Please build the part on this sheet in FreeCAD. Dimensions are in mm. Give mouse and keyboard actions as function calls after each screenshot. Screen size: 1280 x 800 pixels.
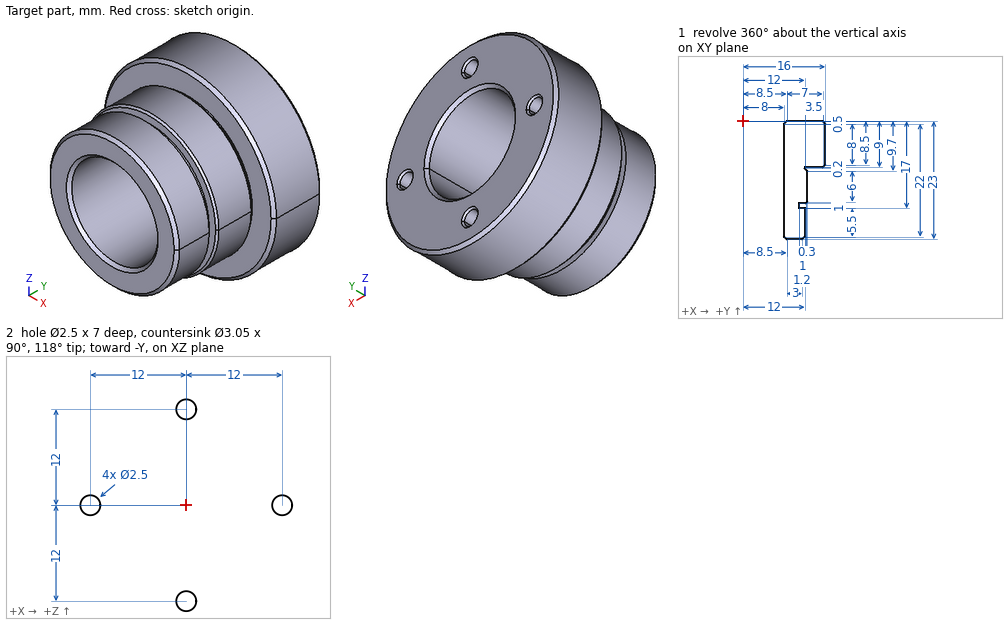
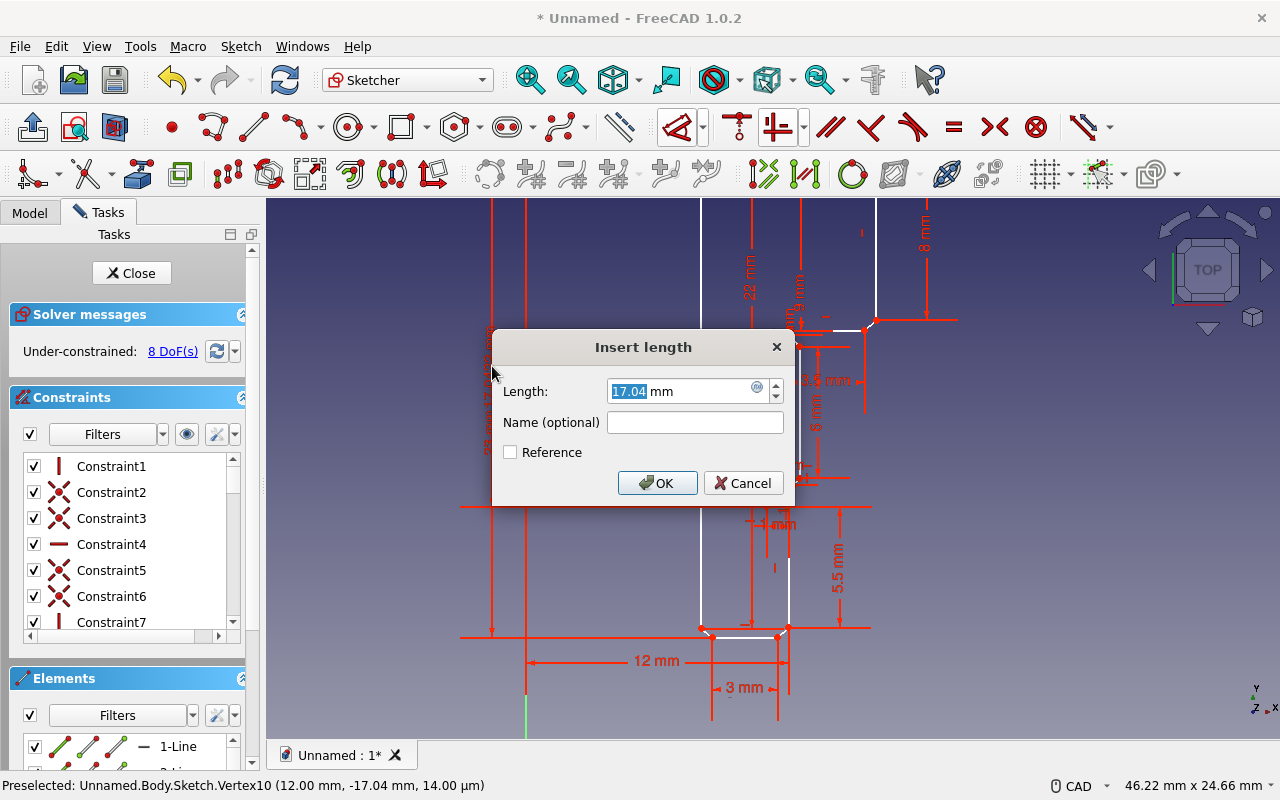
text(17)
key(Return)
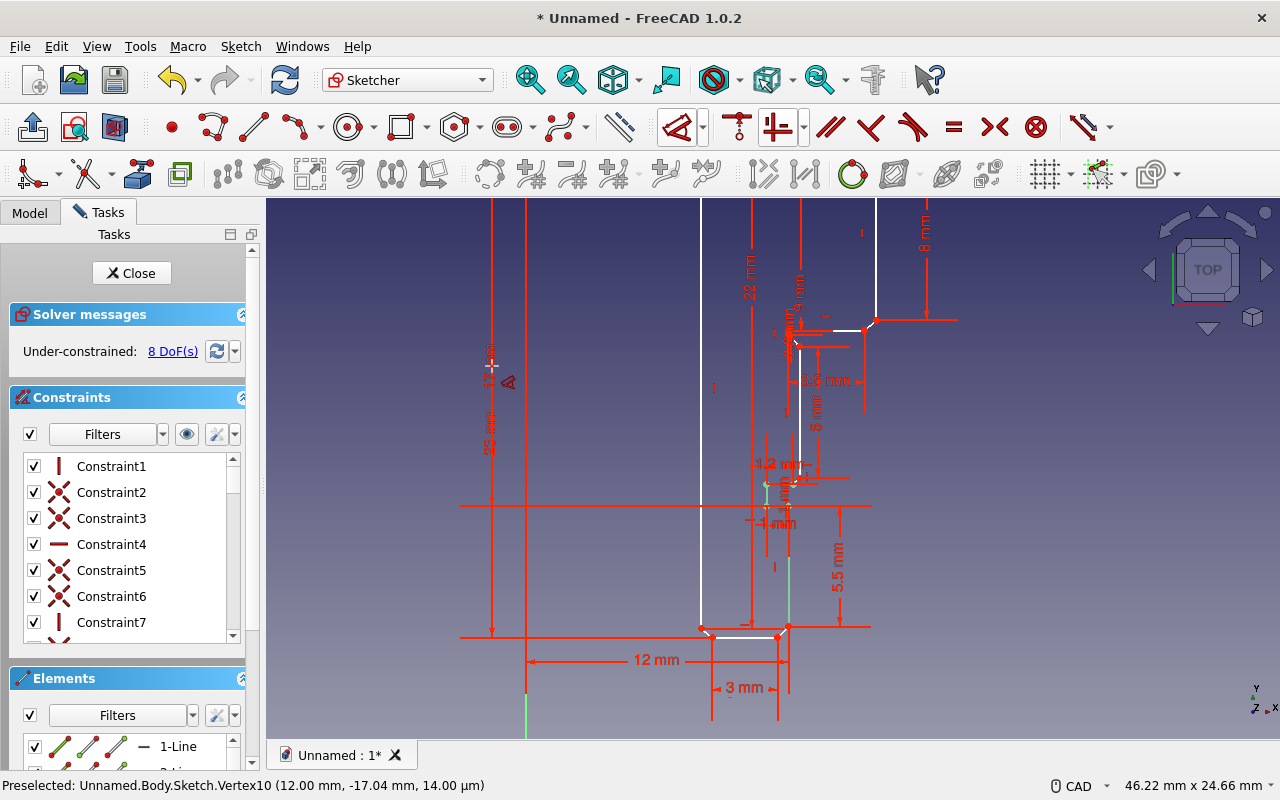
scroll(788, 335, up, 6)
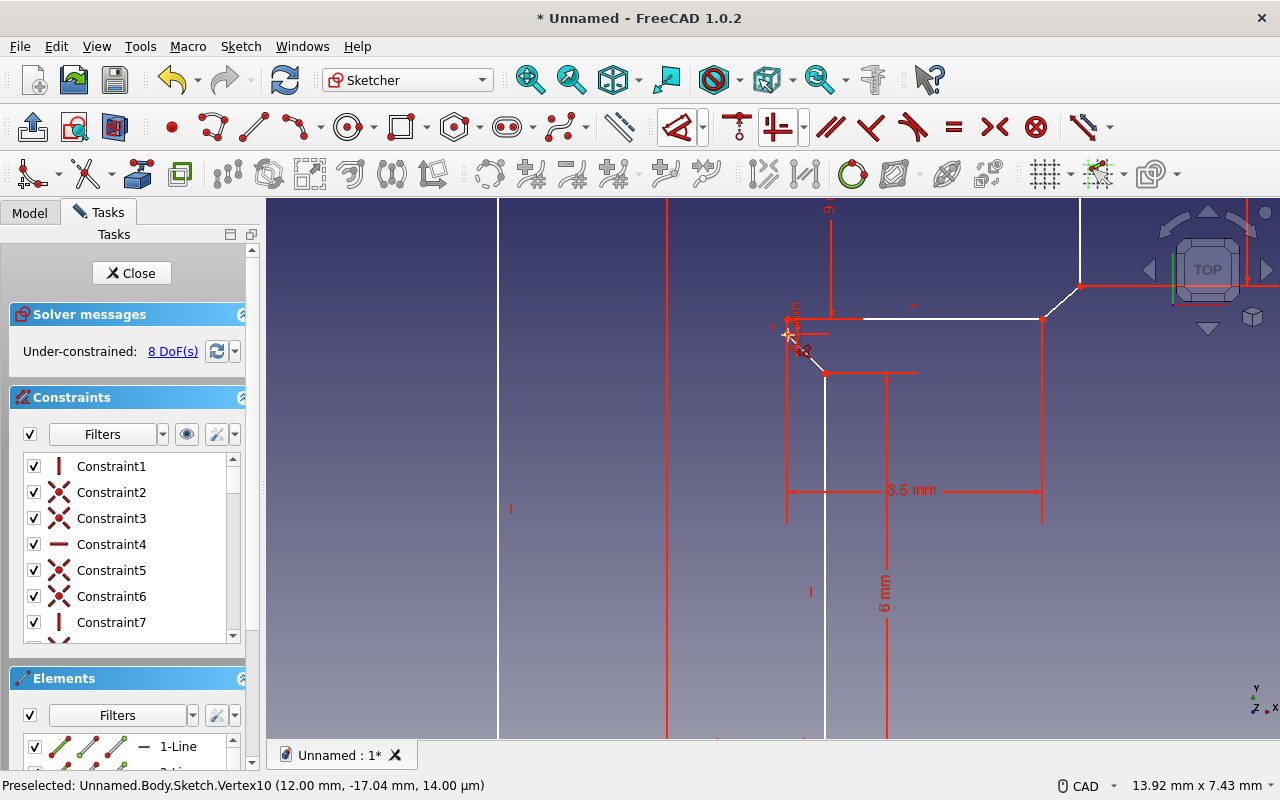
click(787, 334)
click(541, 368)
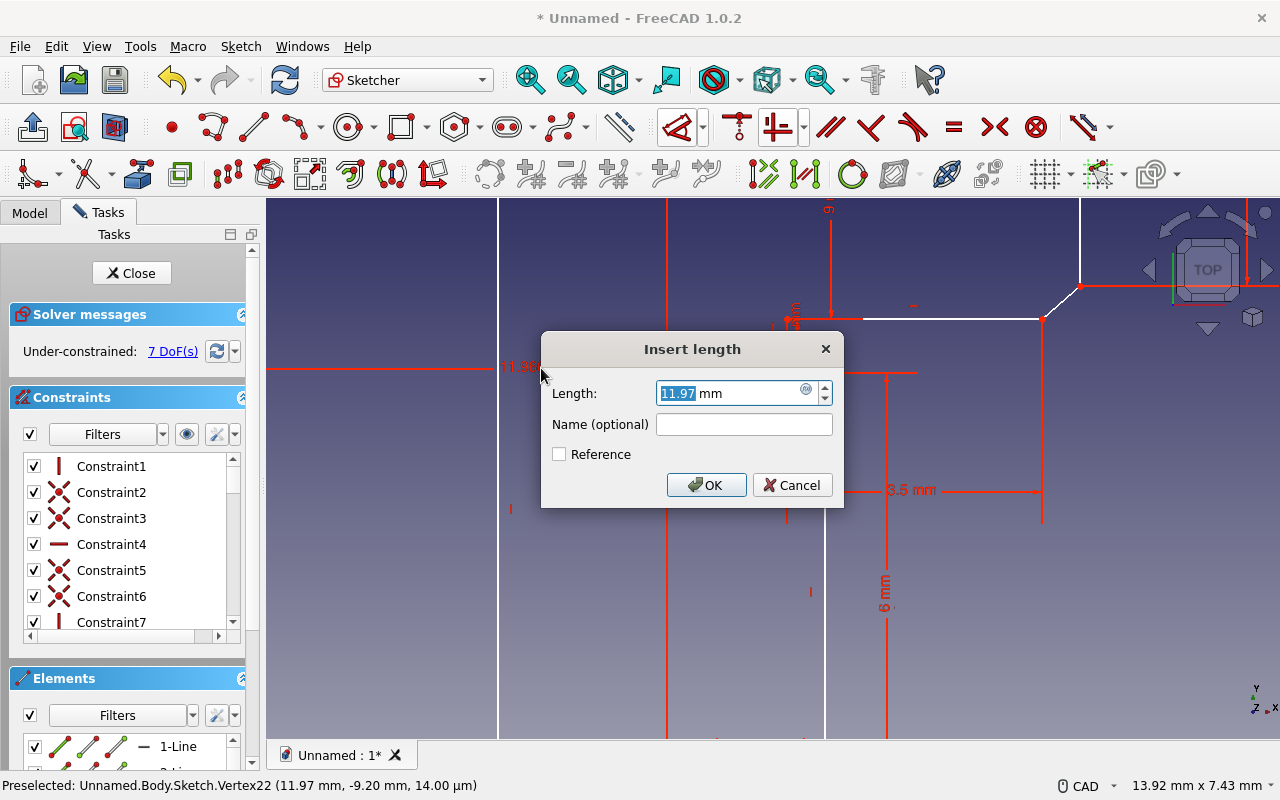
text(12)
key(Return)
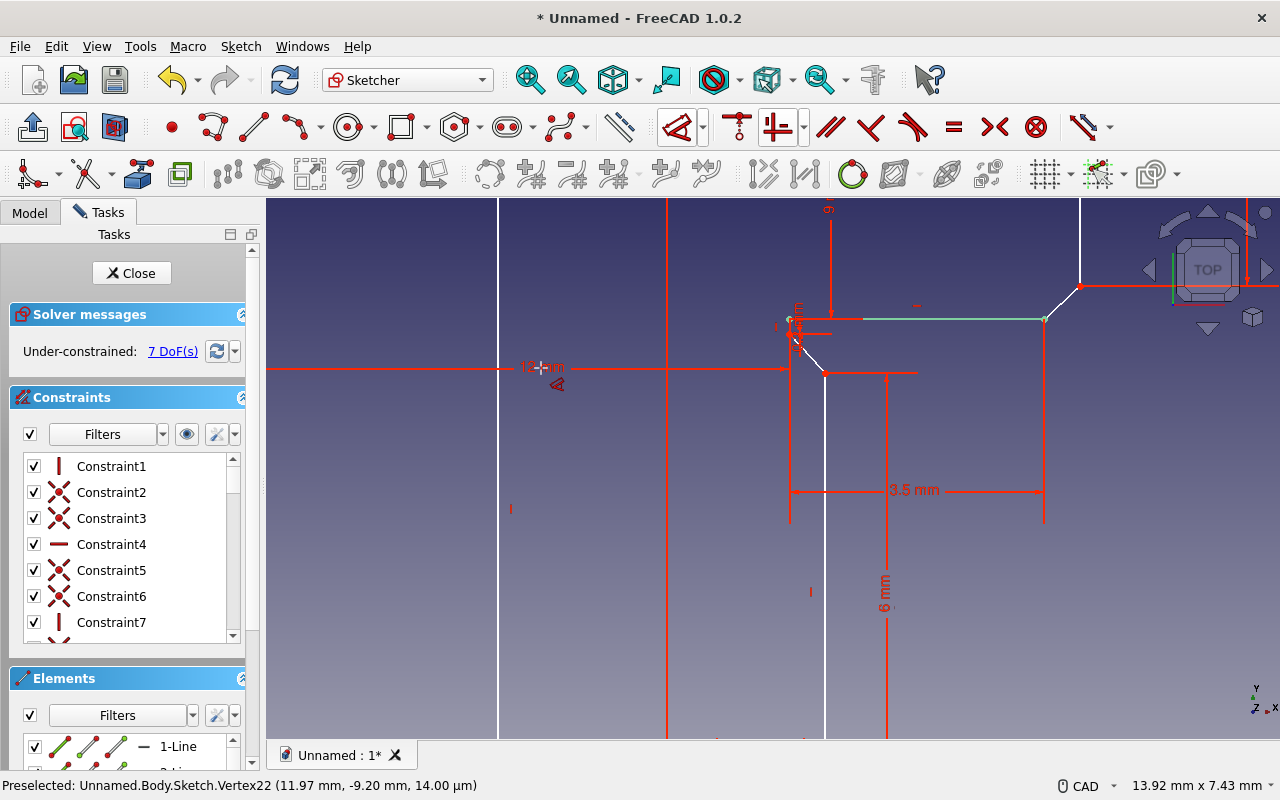
scroll(757, 460, down, 8)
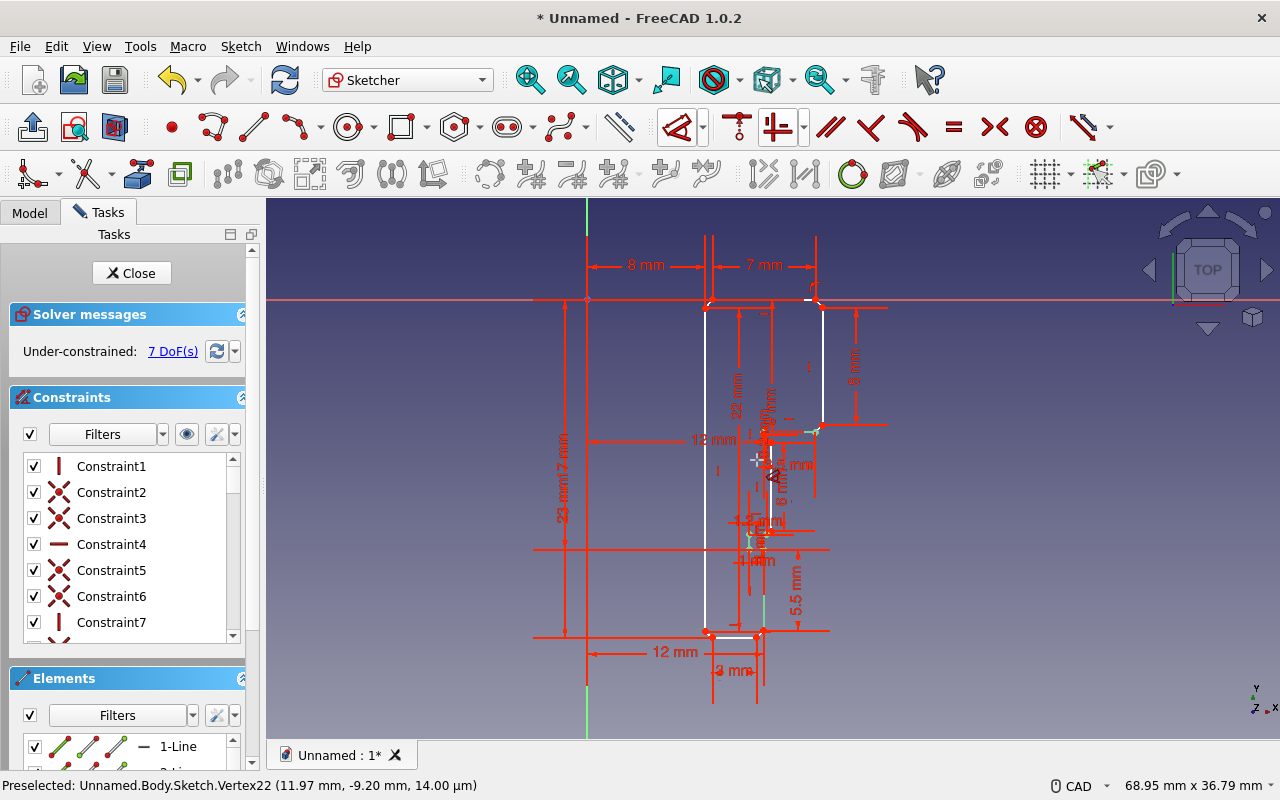
scroll(823, 425, up, 2)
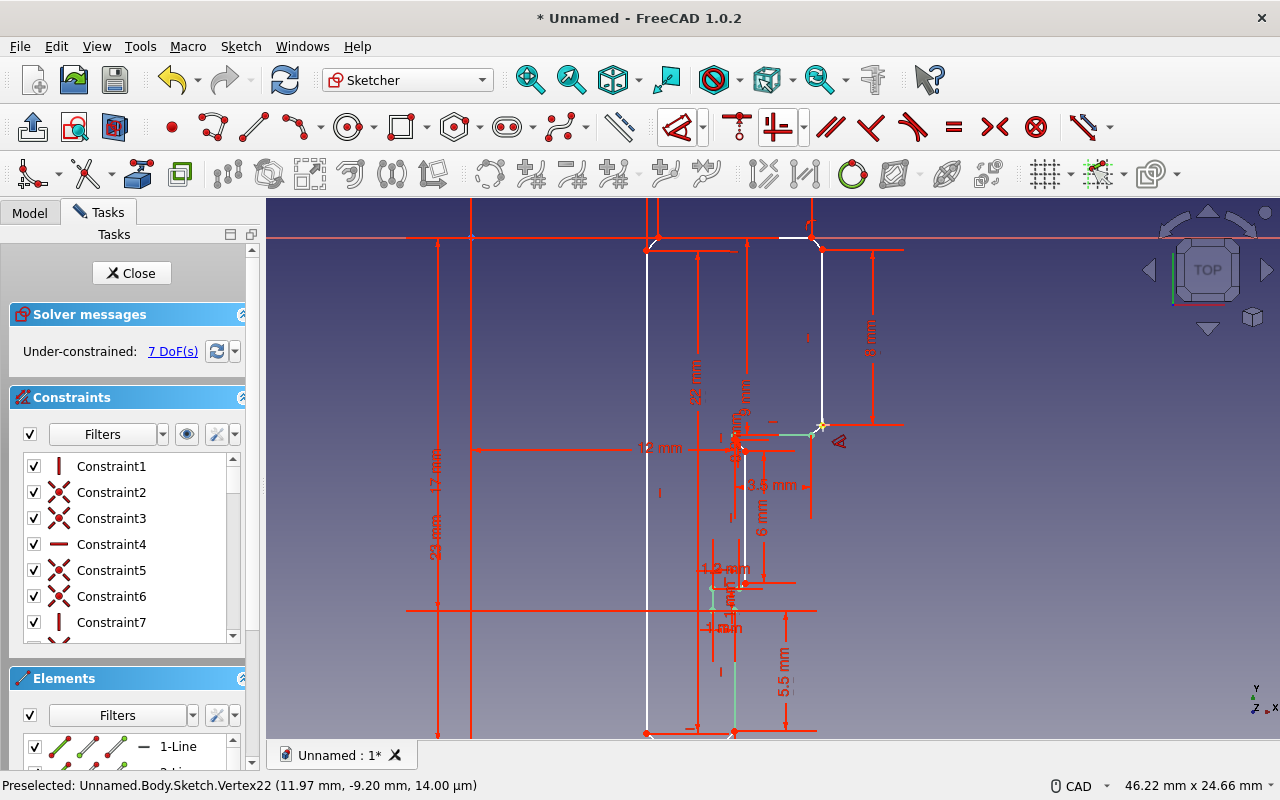
click(822, 425)
click(566, 459)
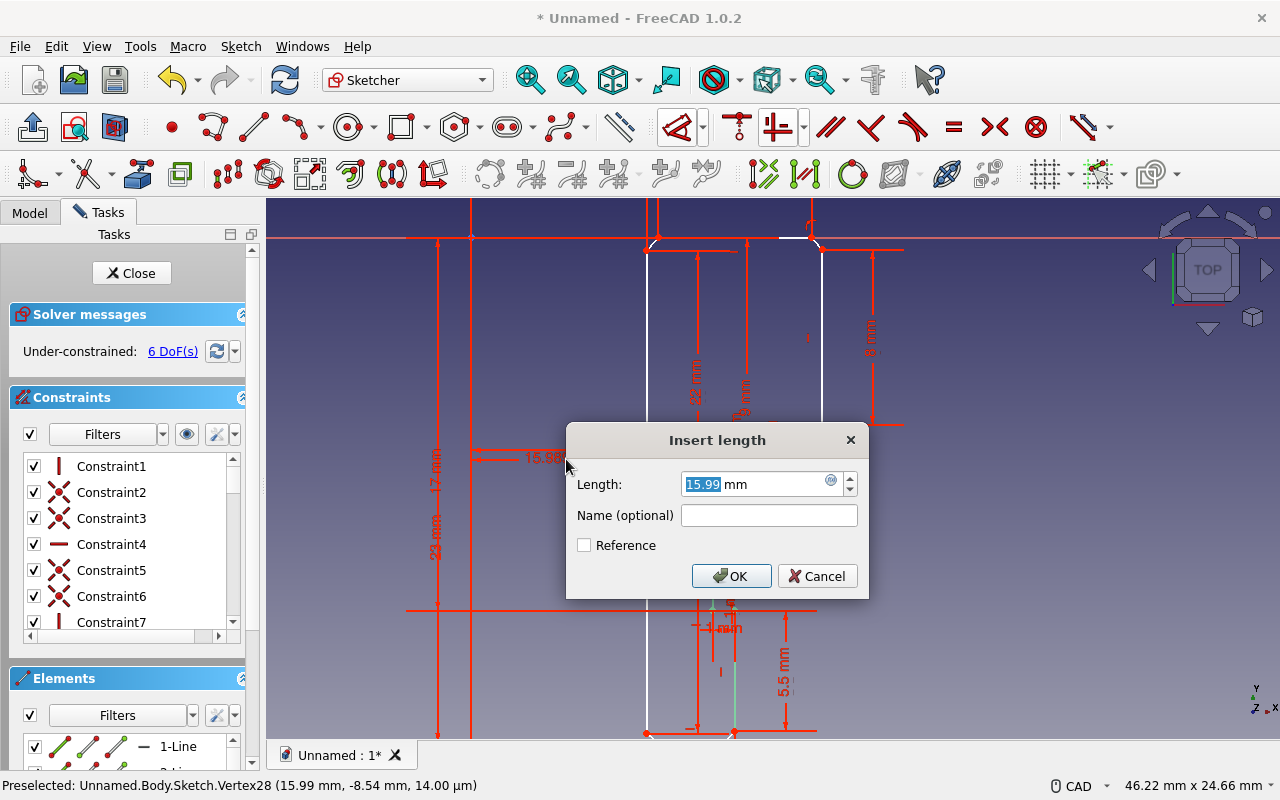
text(16)
key(Return)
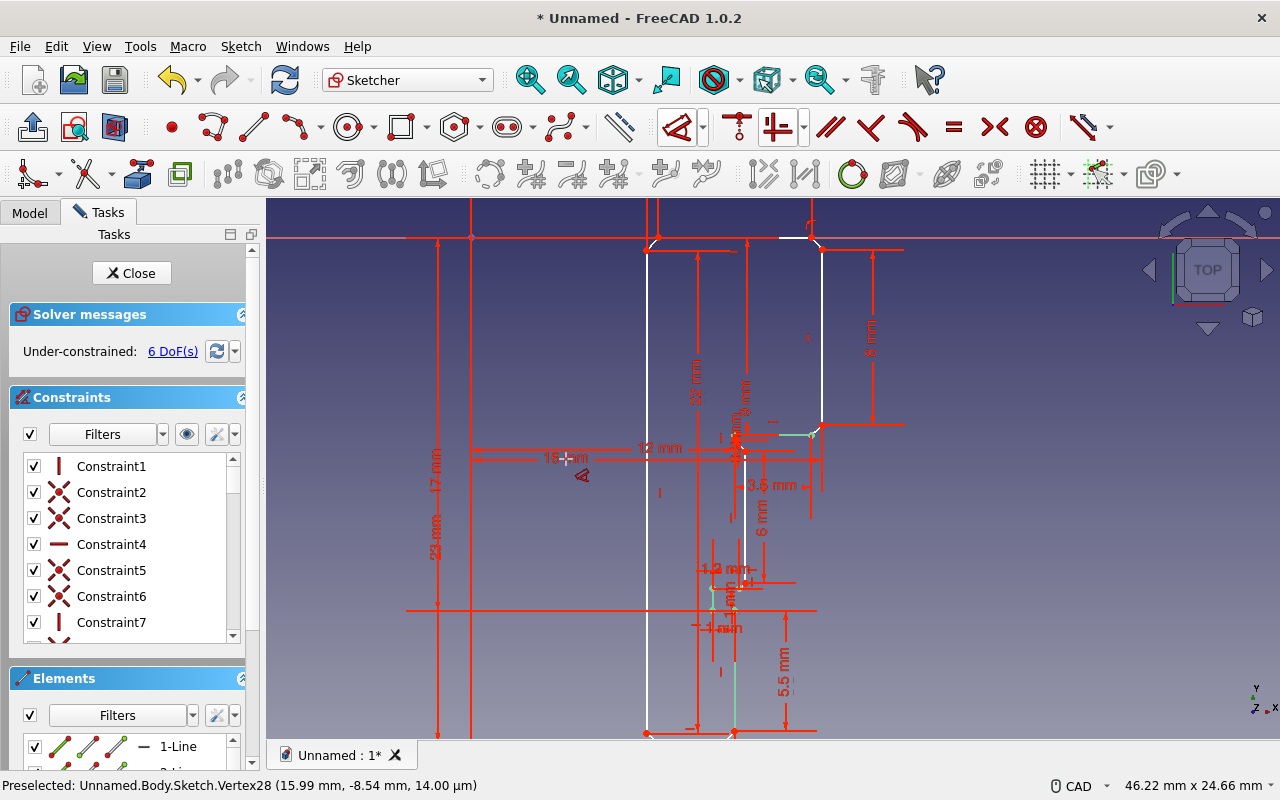
scroll(647, 251, up, 7)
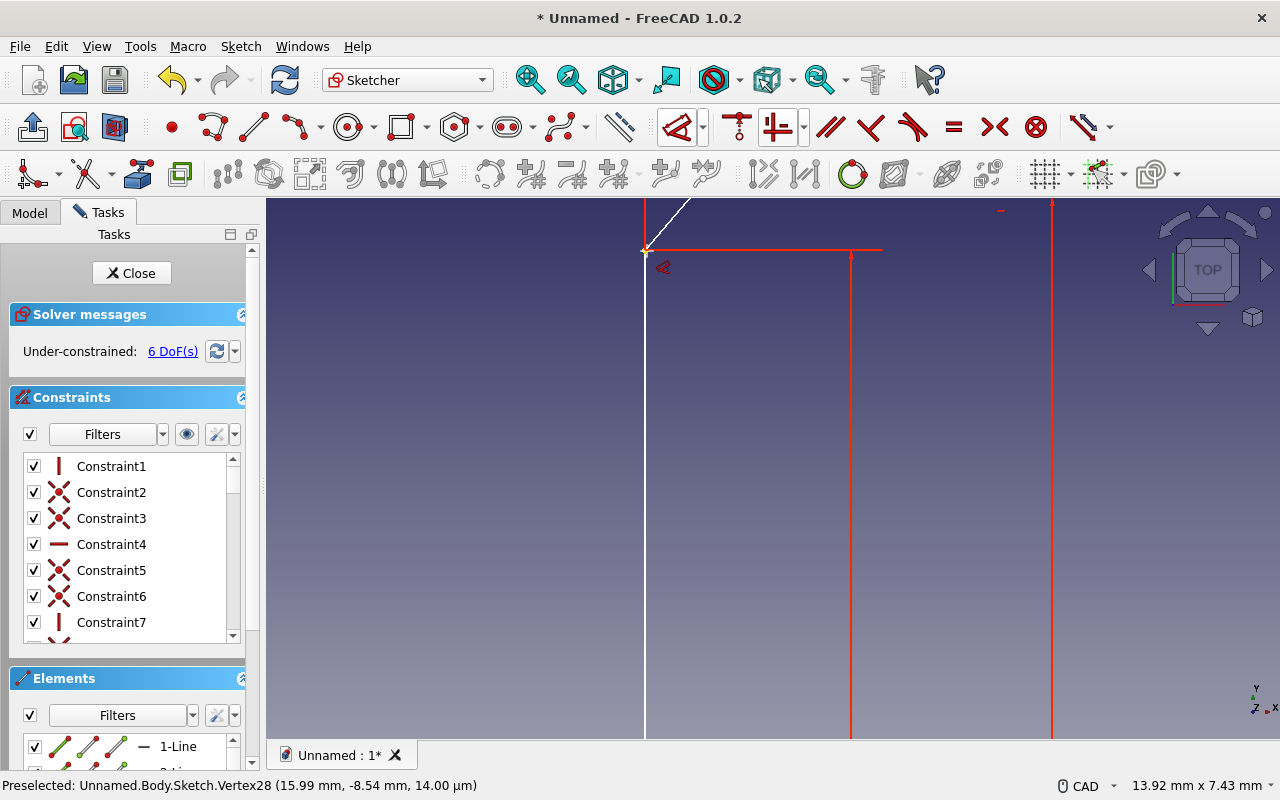
click(645, 250)
click(679, 238)